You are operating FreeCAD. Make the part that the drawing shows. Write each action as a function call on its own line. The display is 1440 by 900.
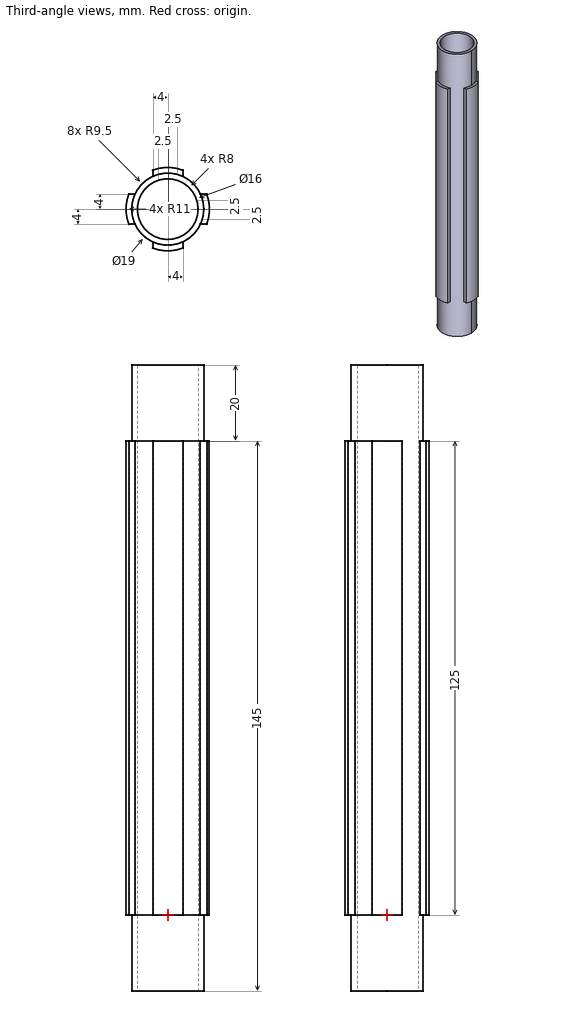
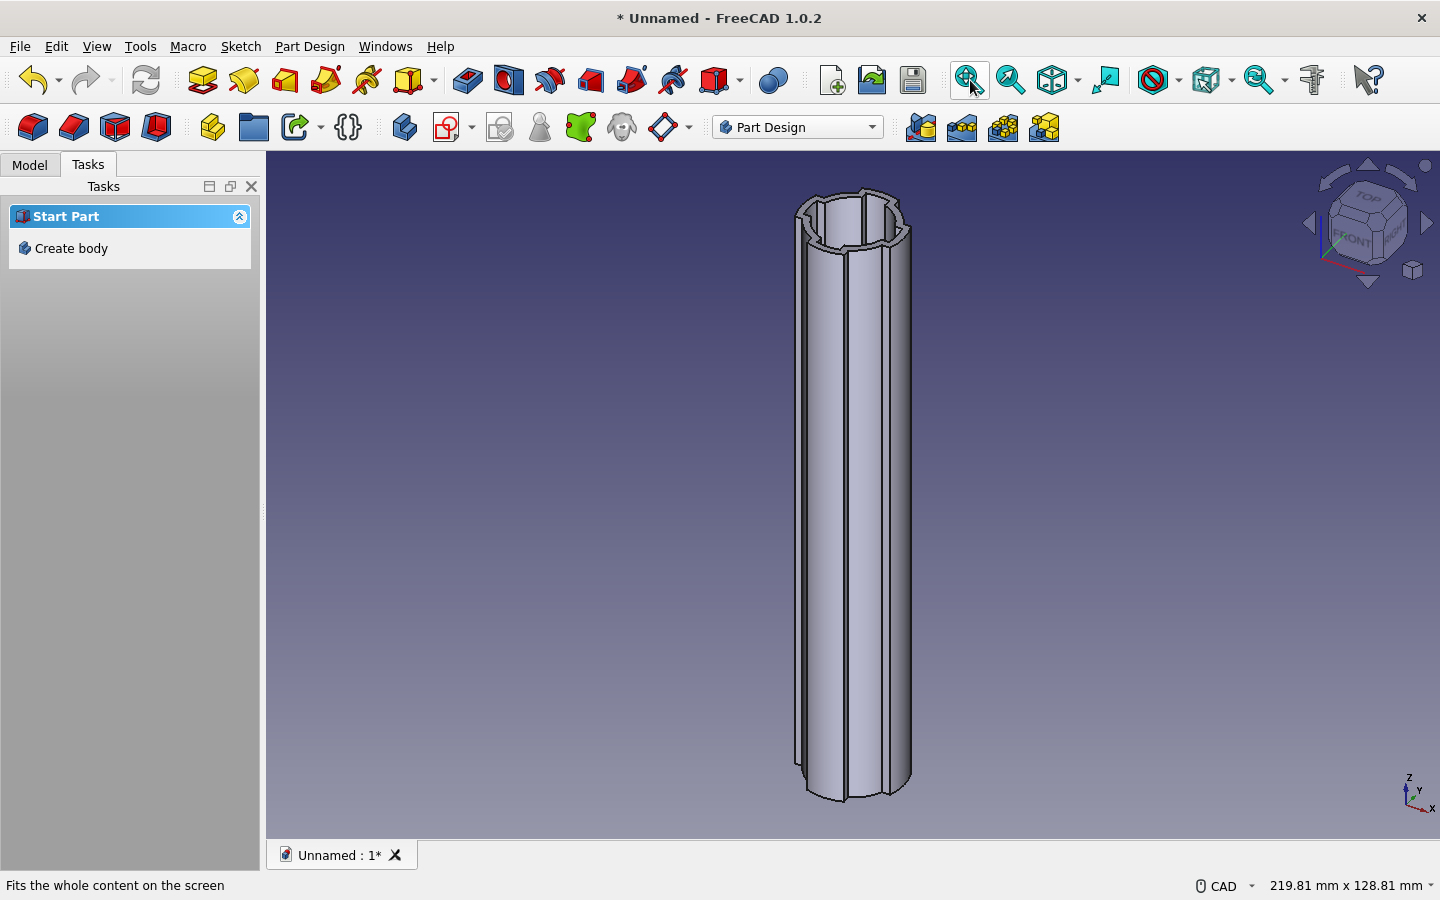
scroll(813, 241, up, 6)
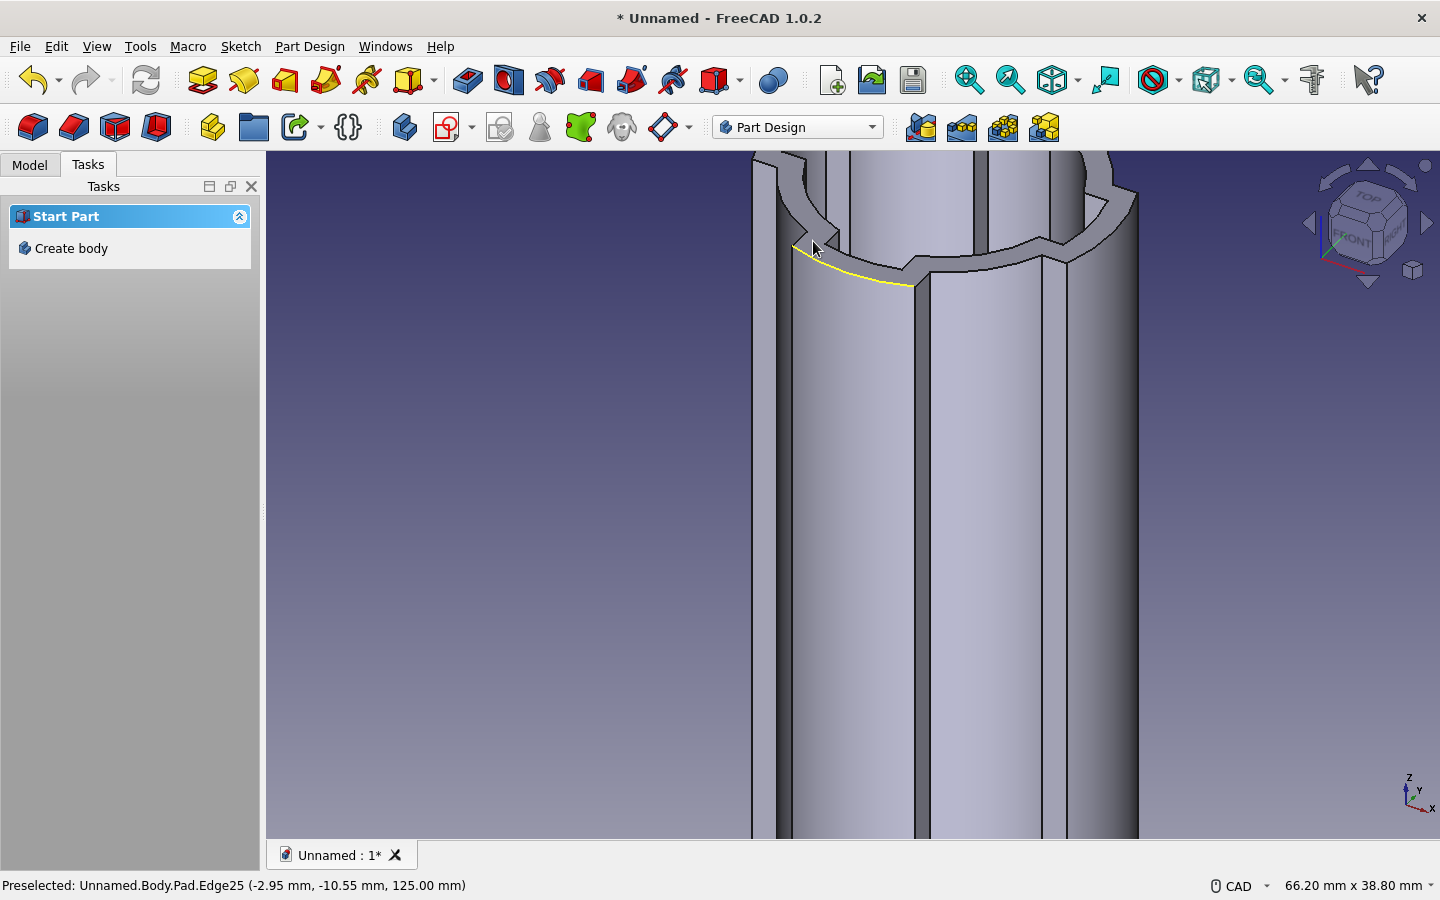
click(813, 242)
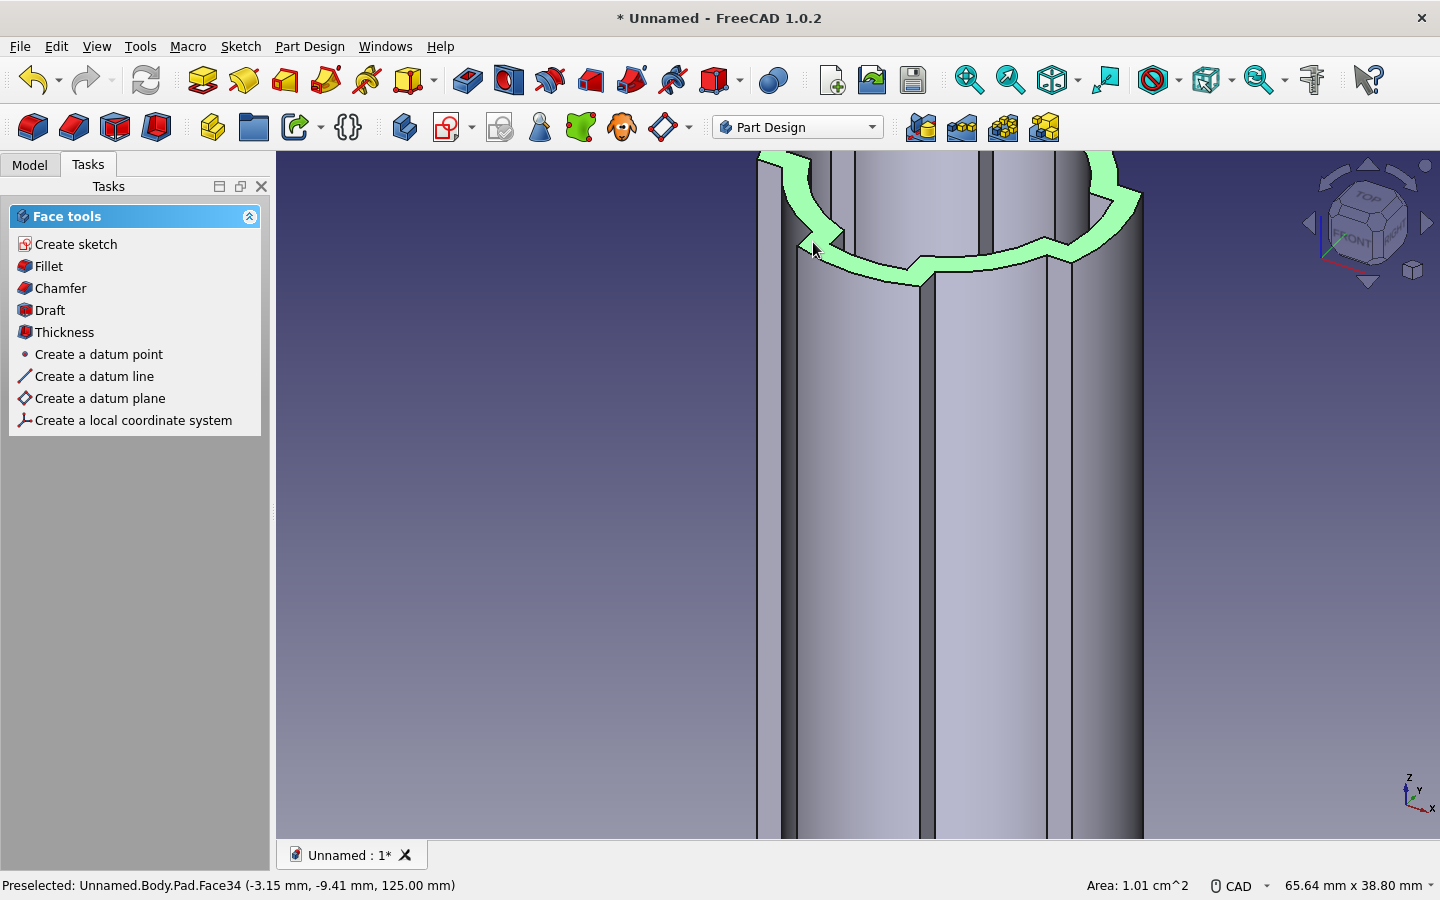
click(446, 128)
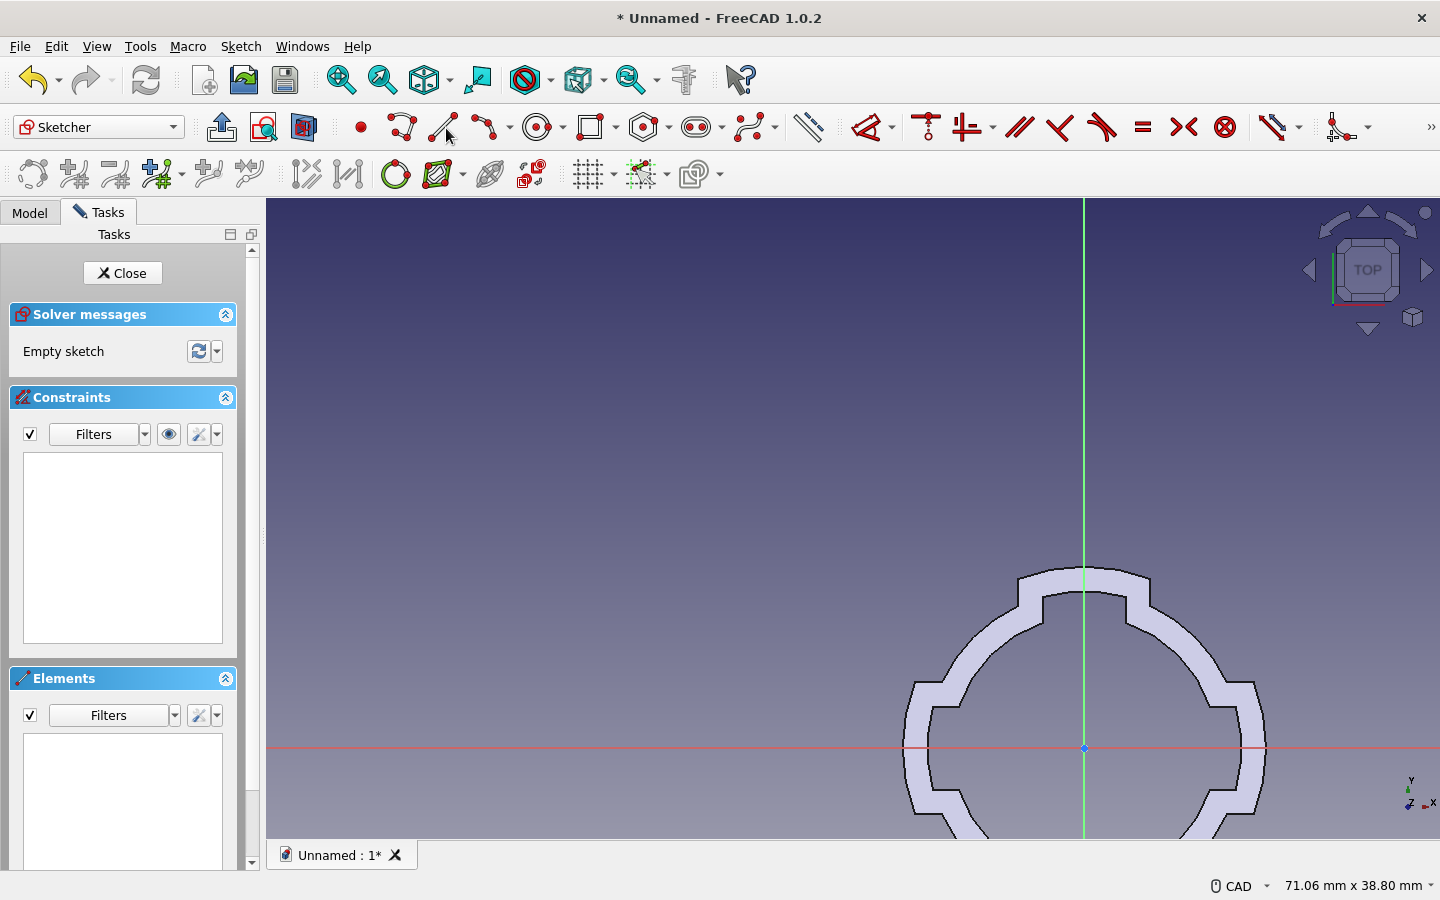
scroll(294, 226, down, 1)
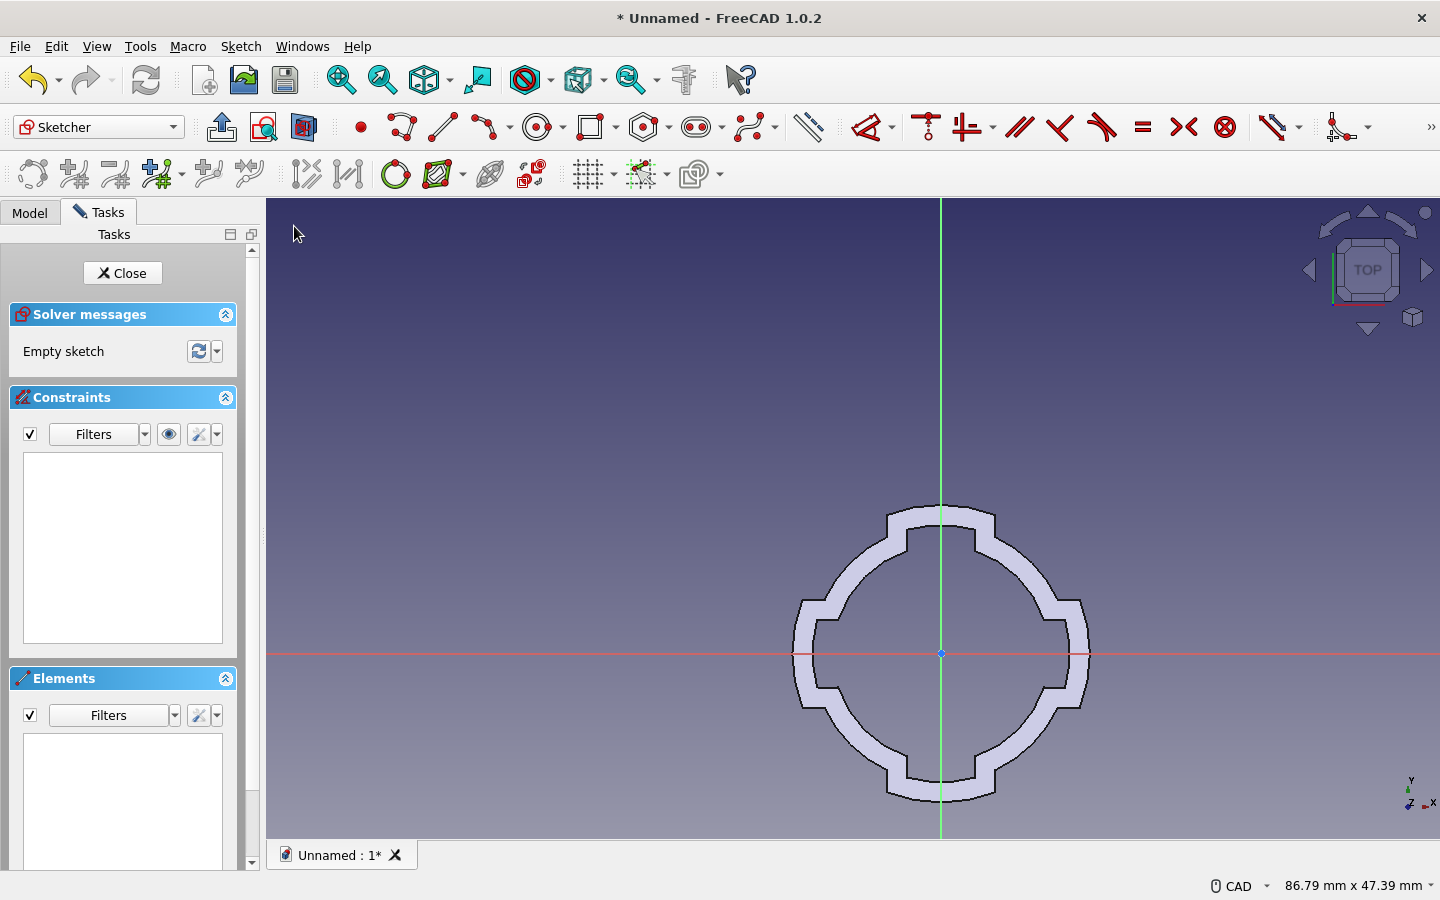
scroll(1260, 811, up, 2)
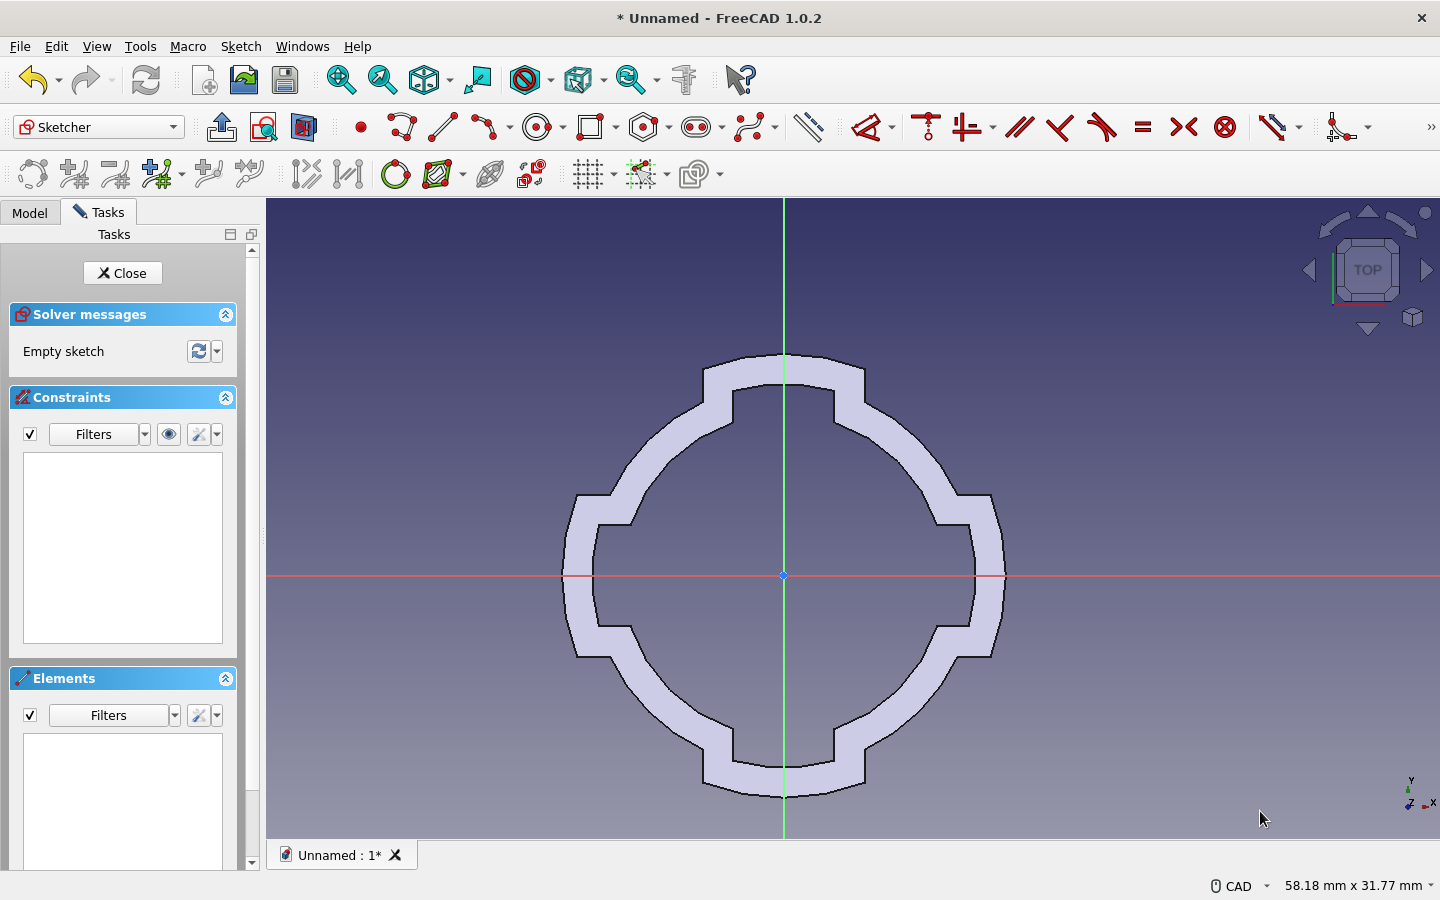
click(536, 128)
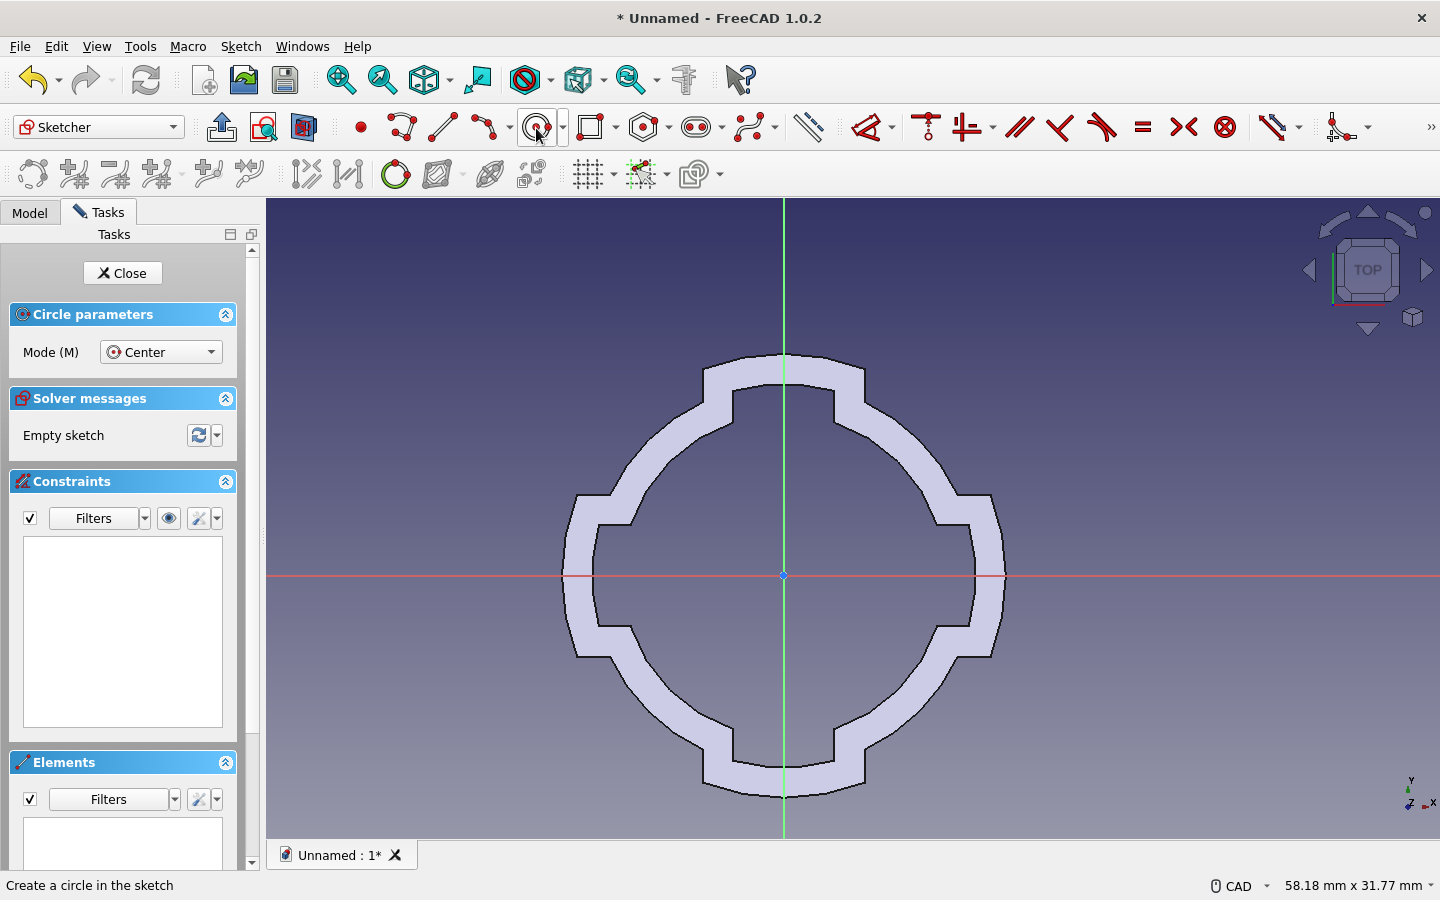
click(784, 576)
move(919, 440)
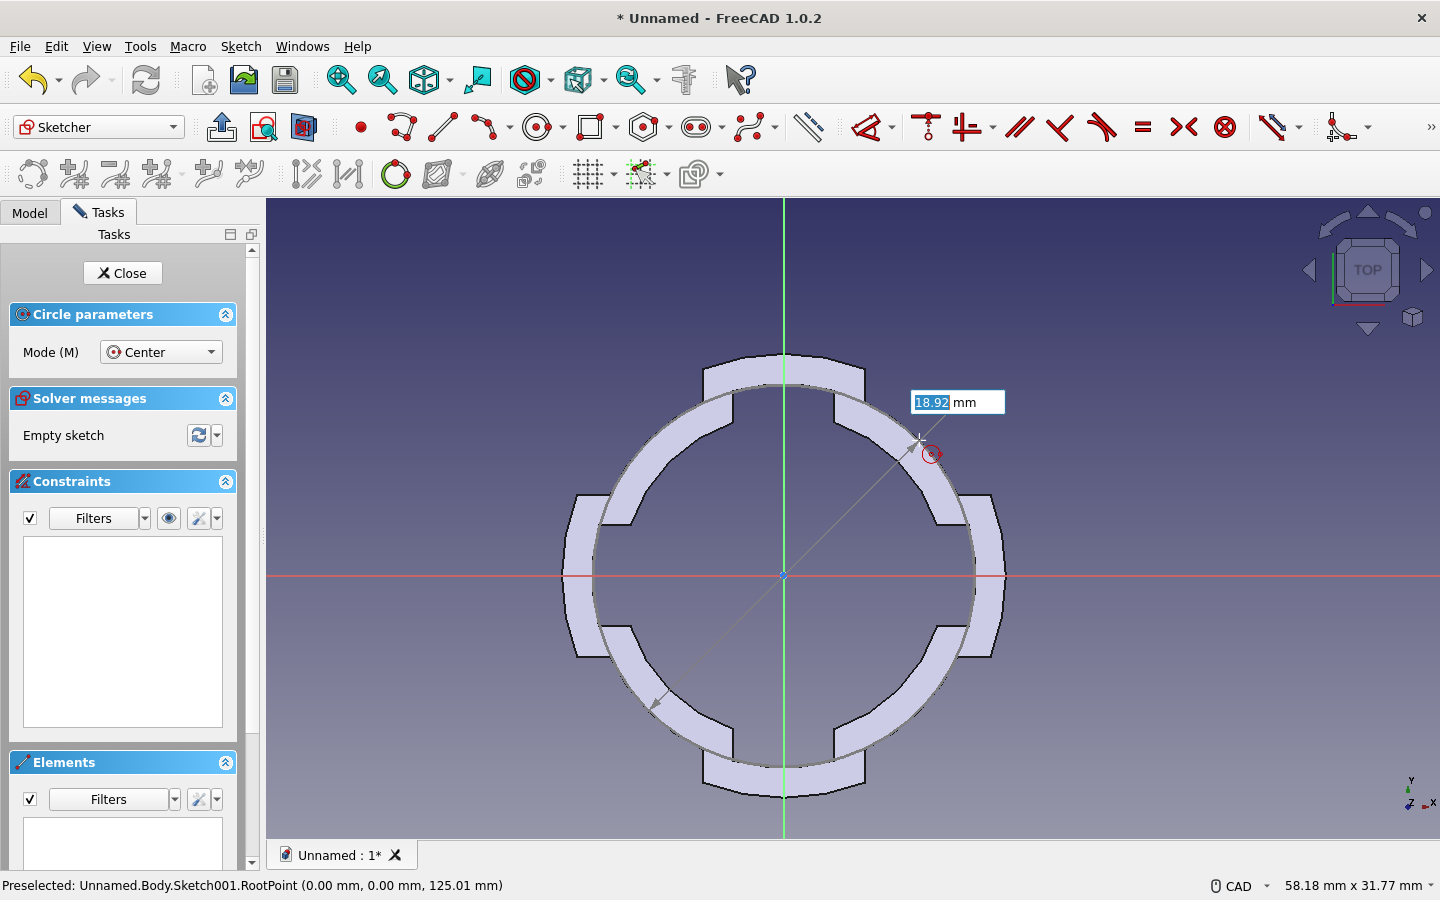
text(19)
key(Return)